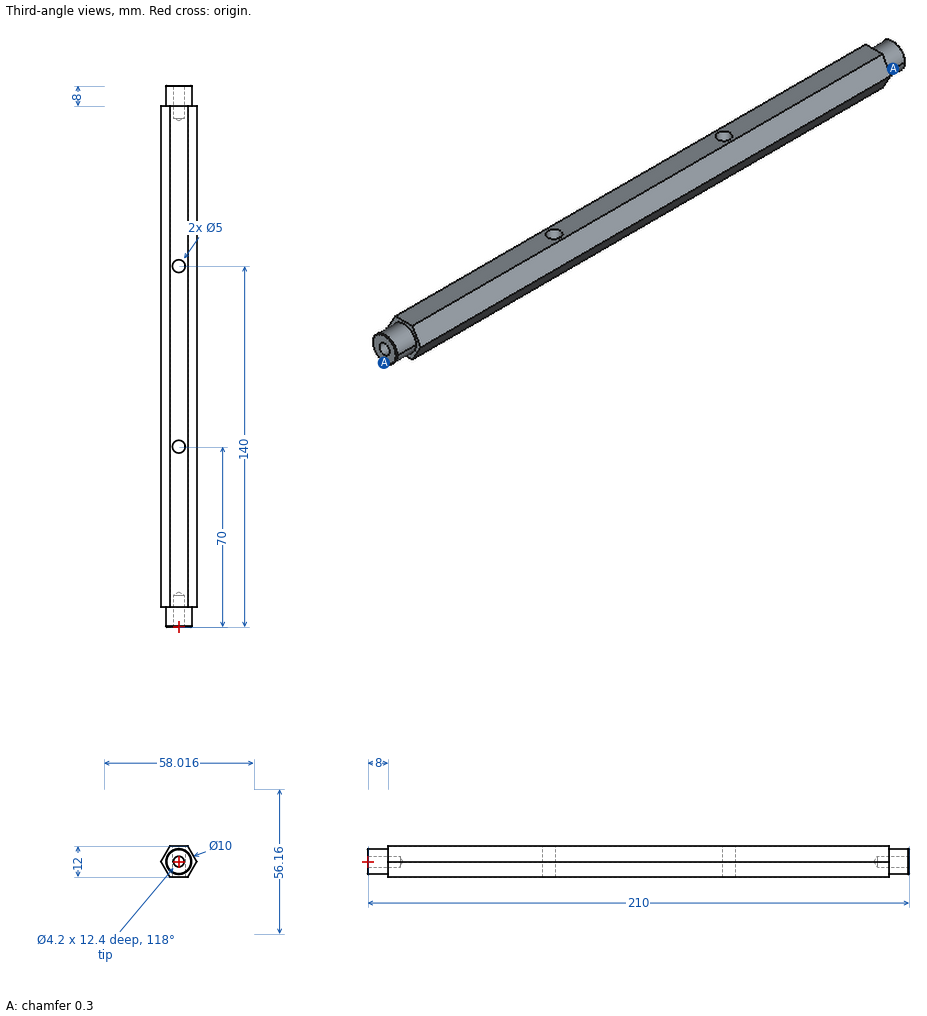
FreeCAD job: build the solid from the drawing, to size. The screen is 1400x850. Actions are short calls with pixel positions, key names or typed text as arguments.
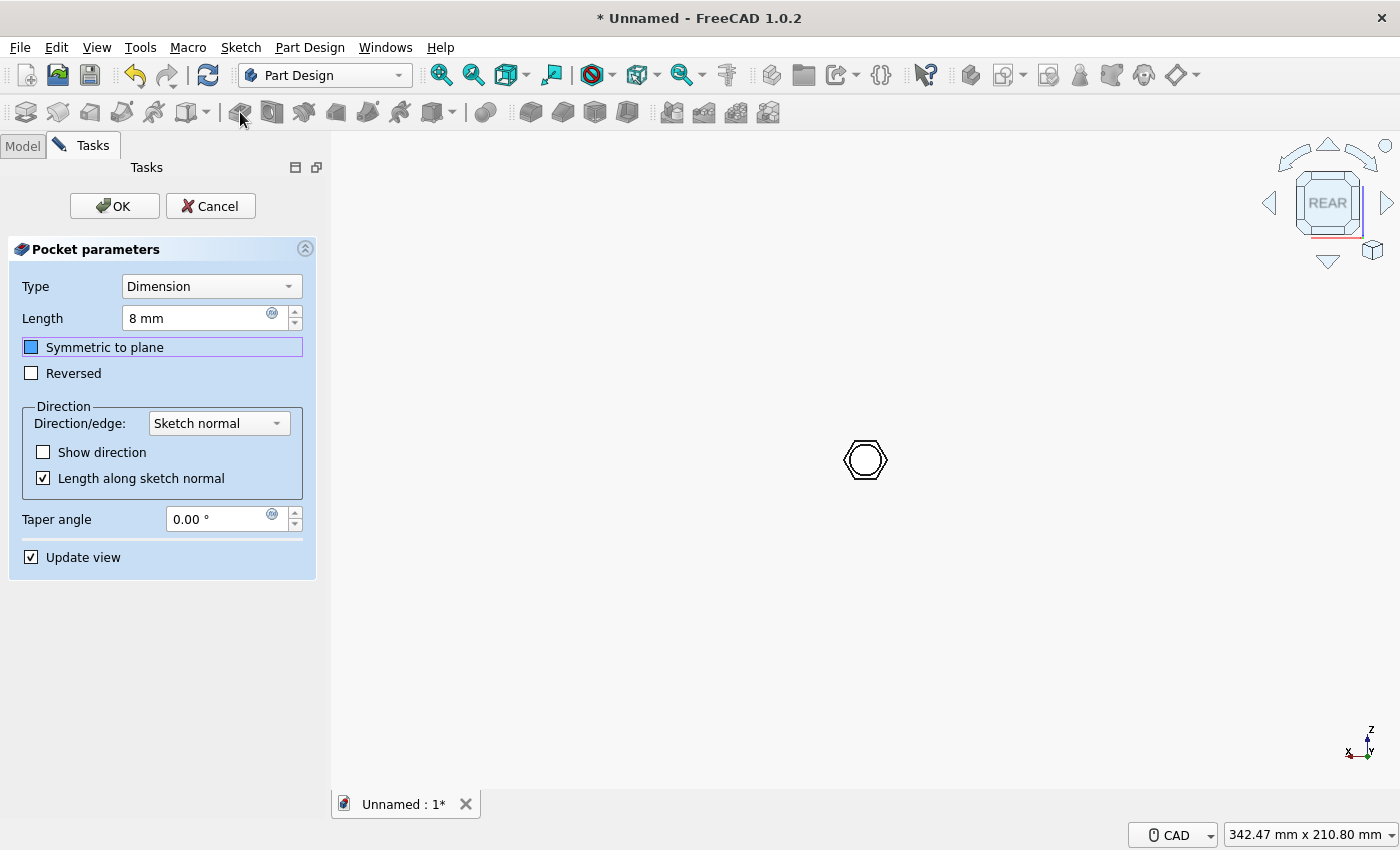
click(115, 206)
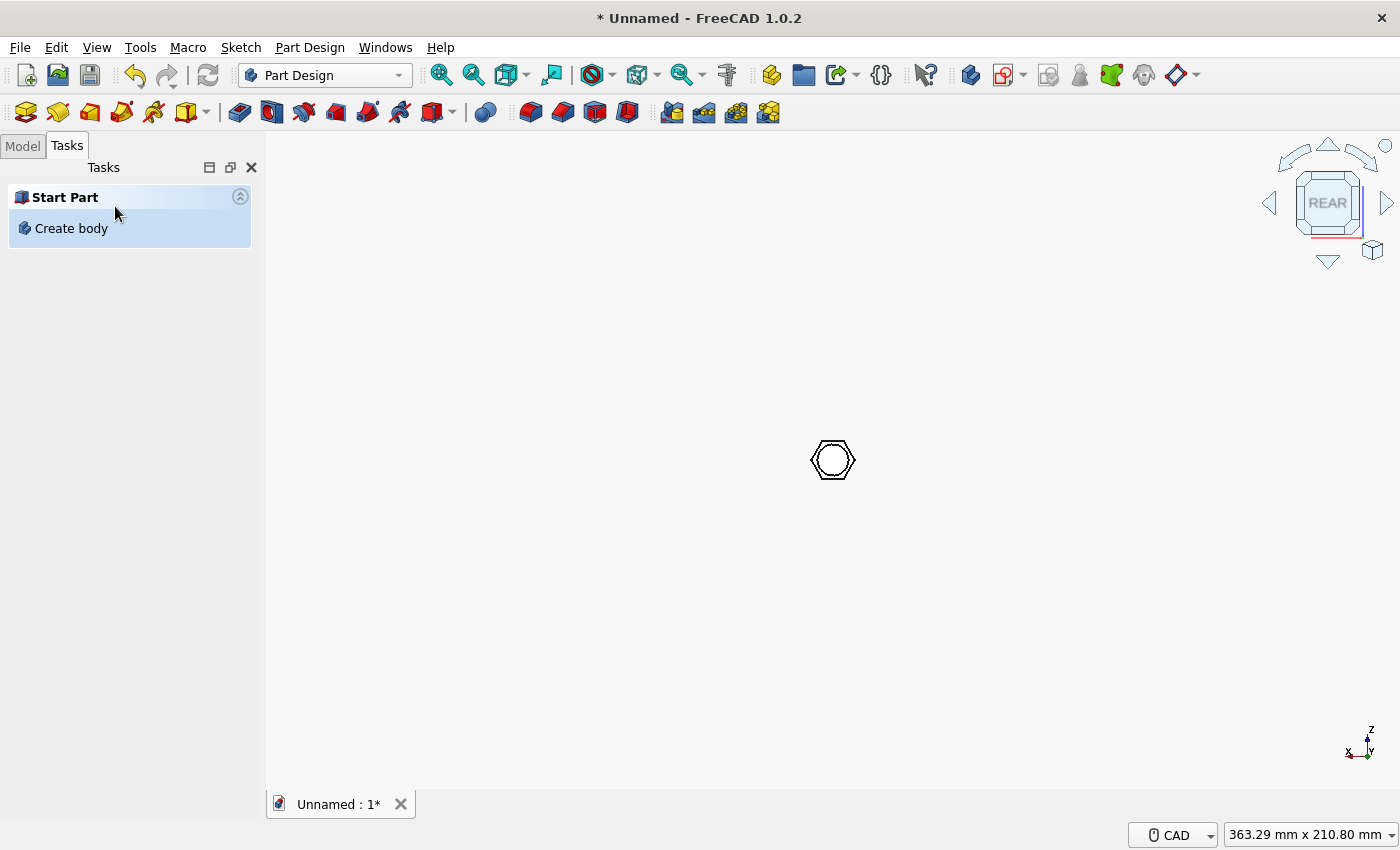
click(442, 76)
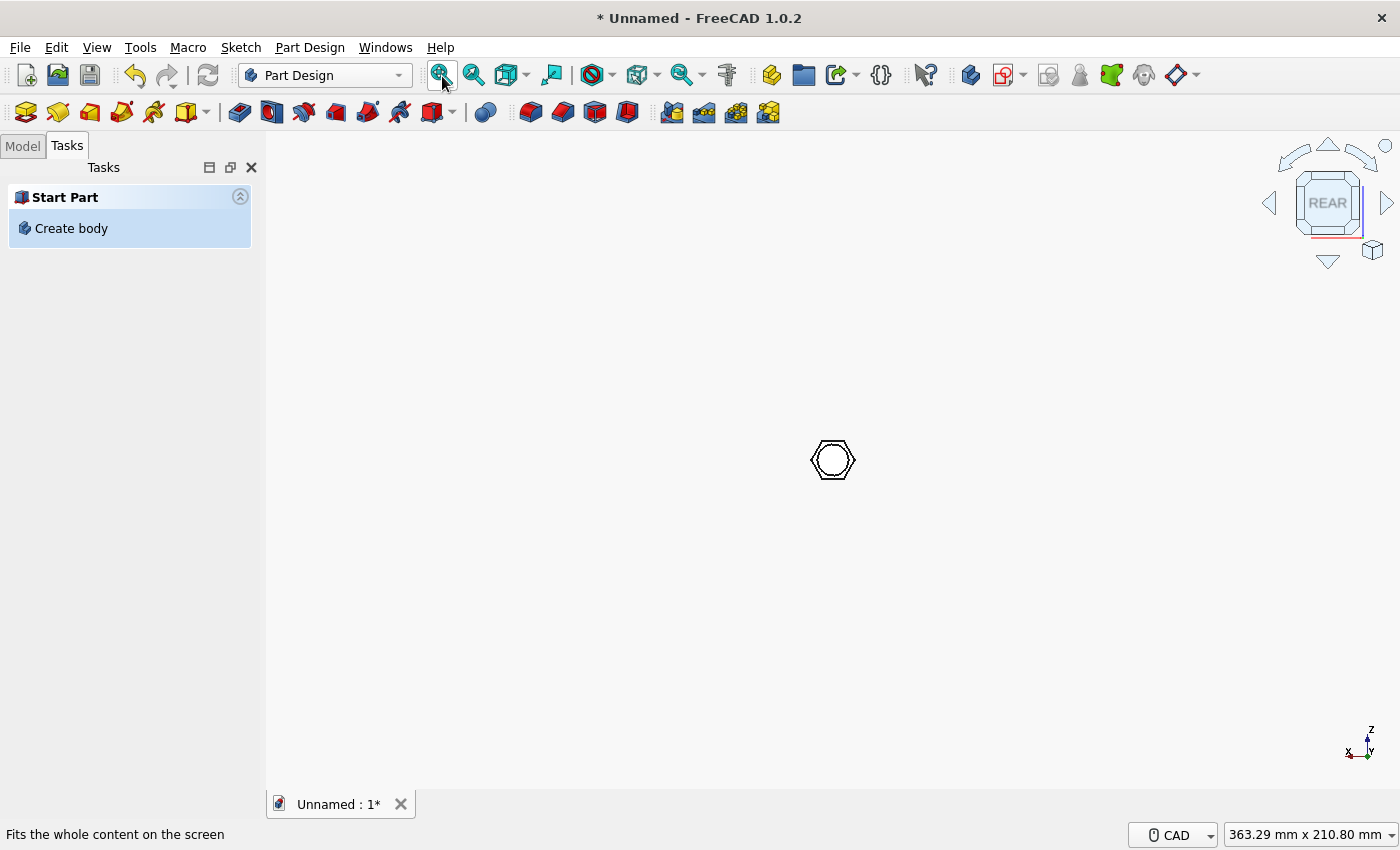
click(1004, 76)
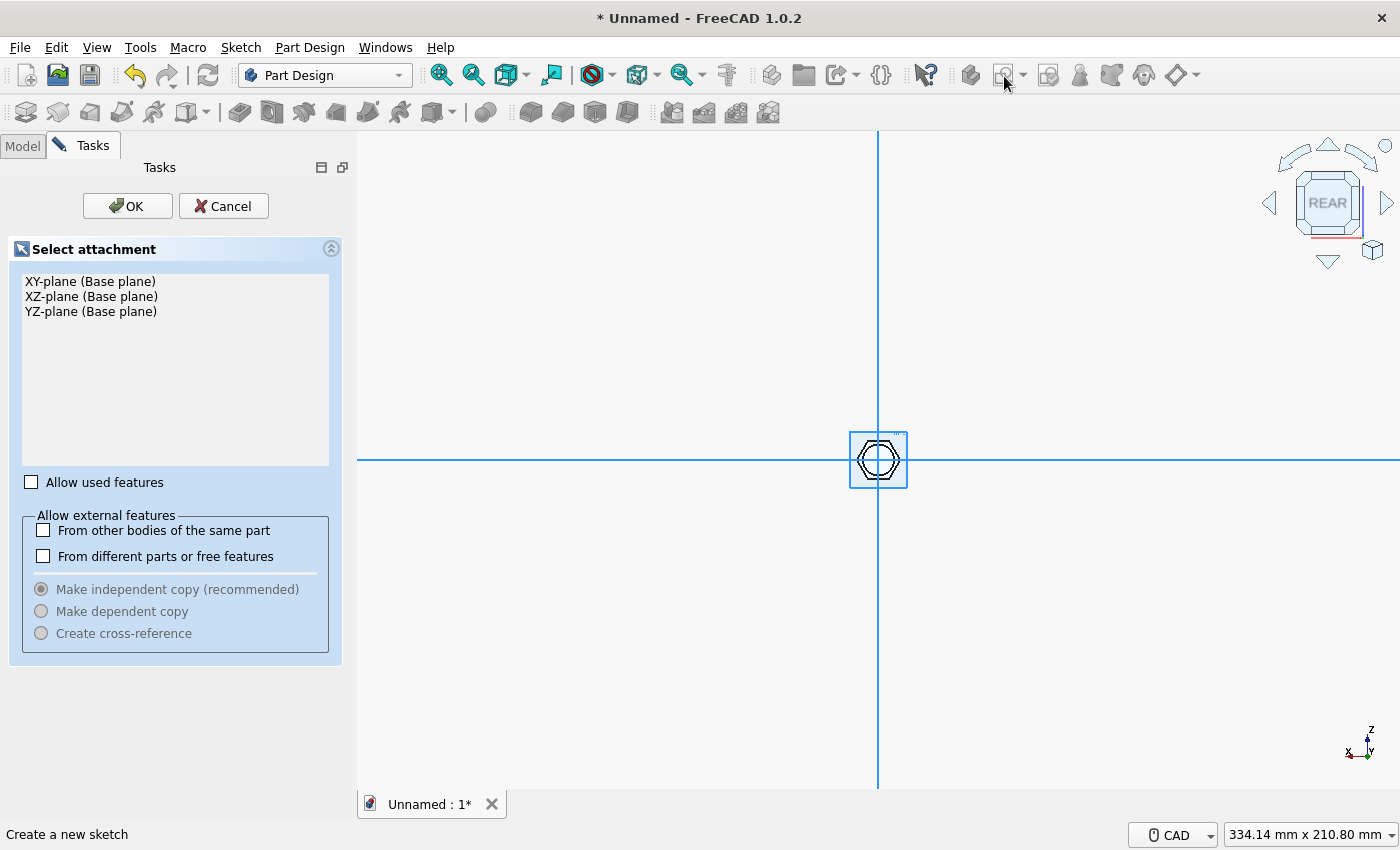
click(82, 296)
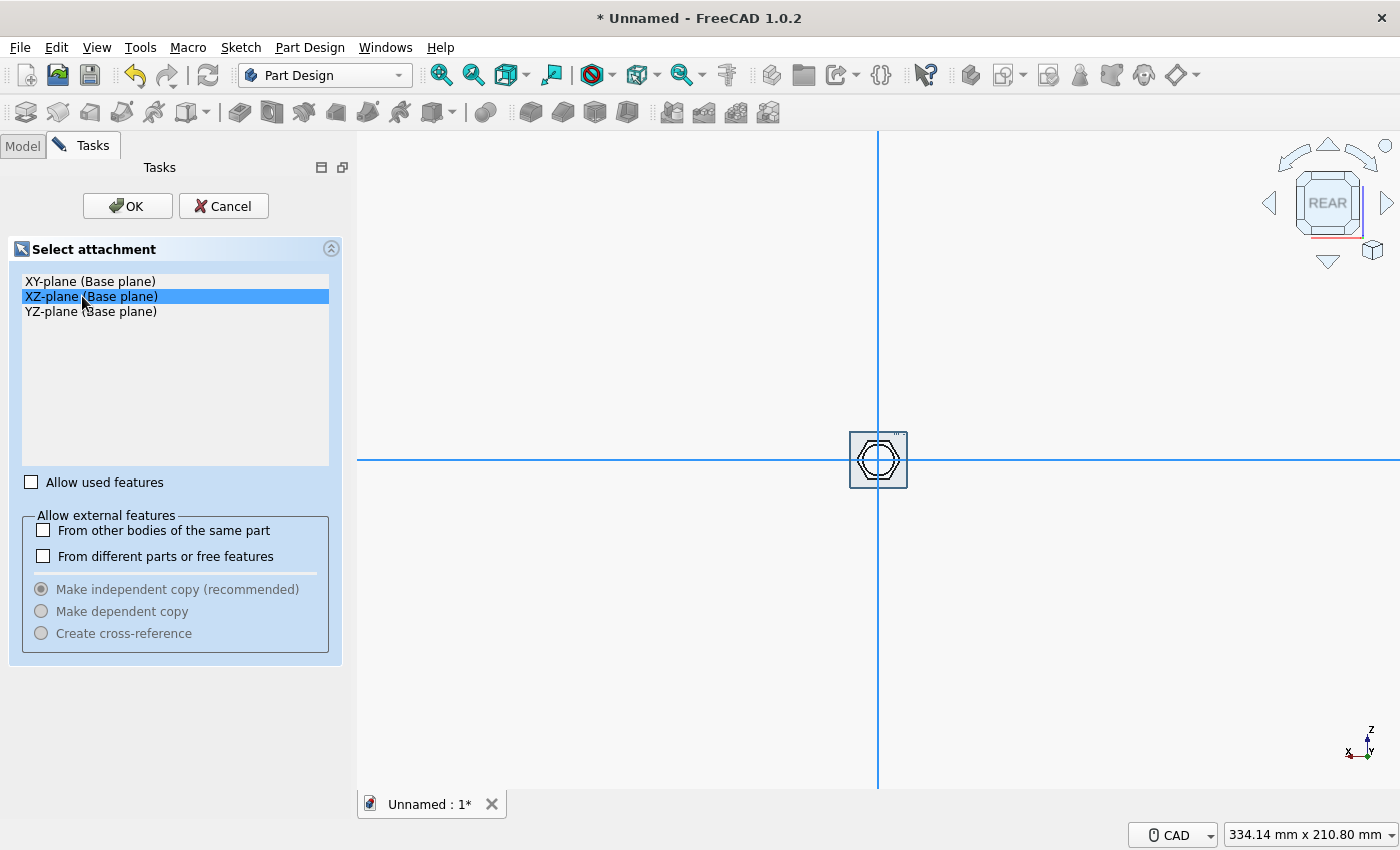
click(128, 206)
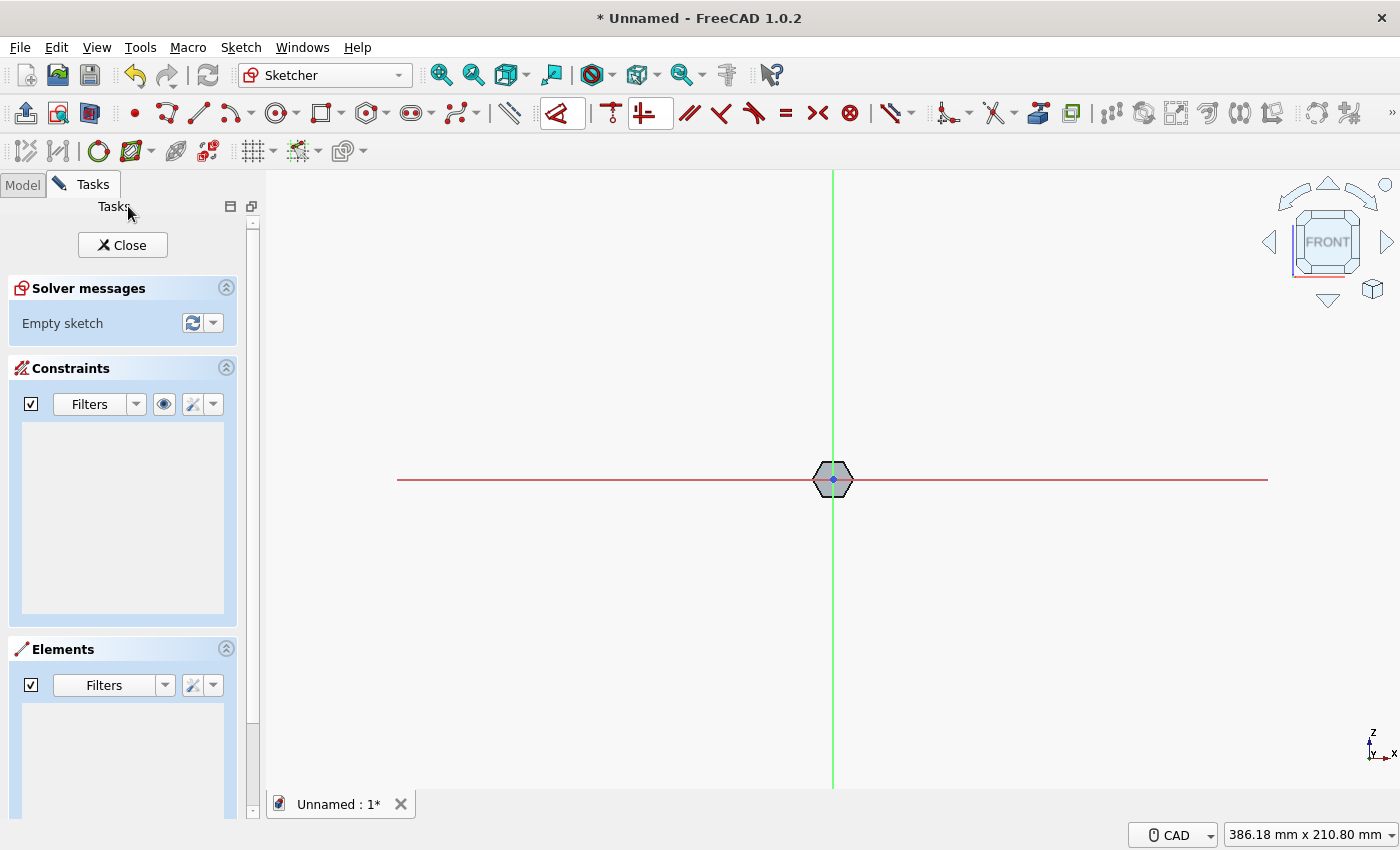
scroll(889, 480, up, 4)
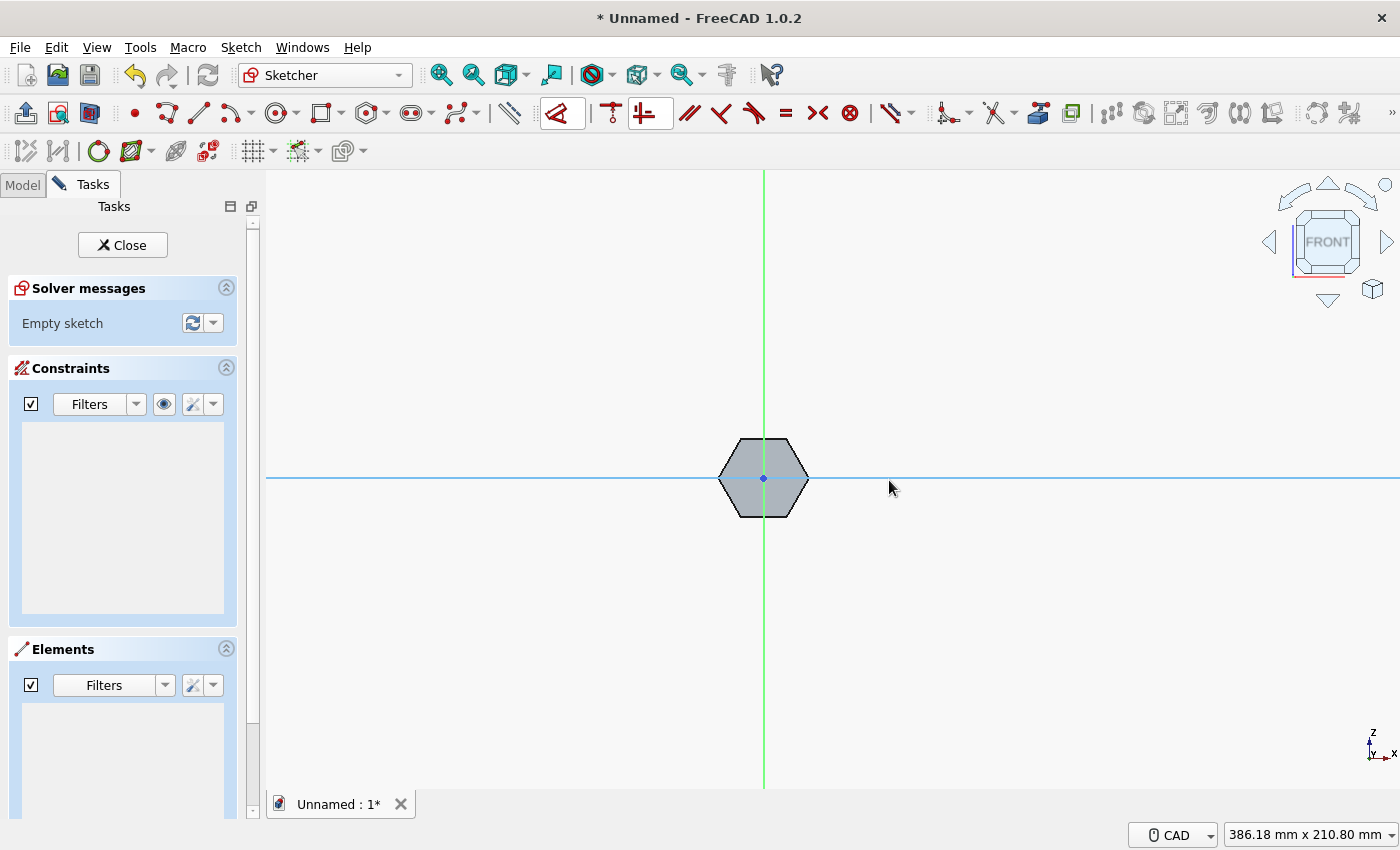
key(g)
key(v)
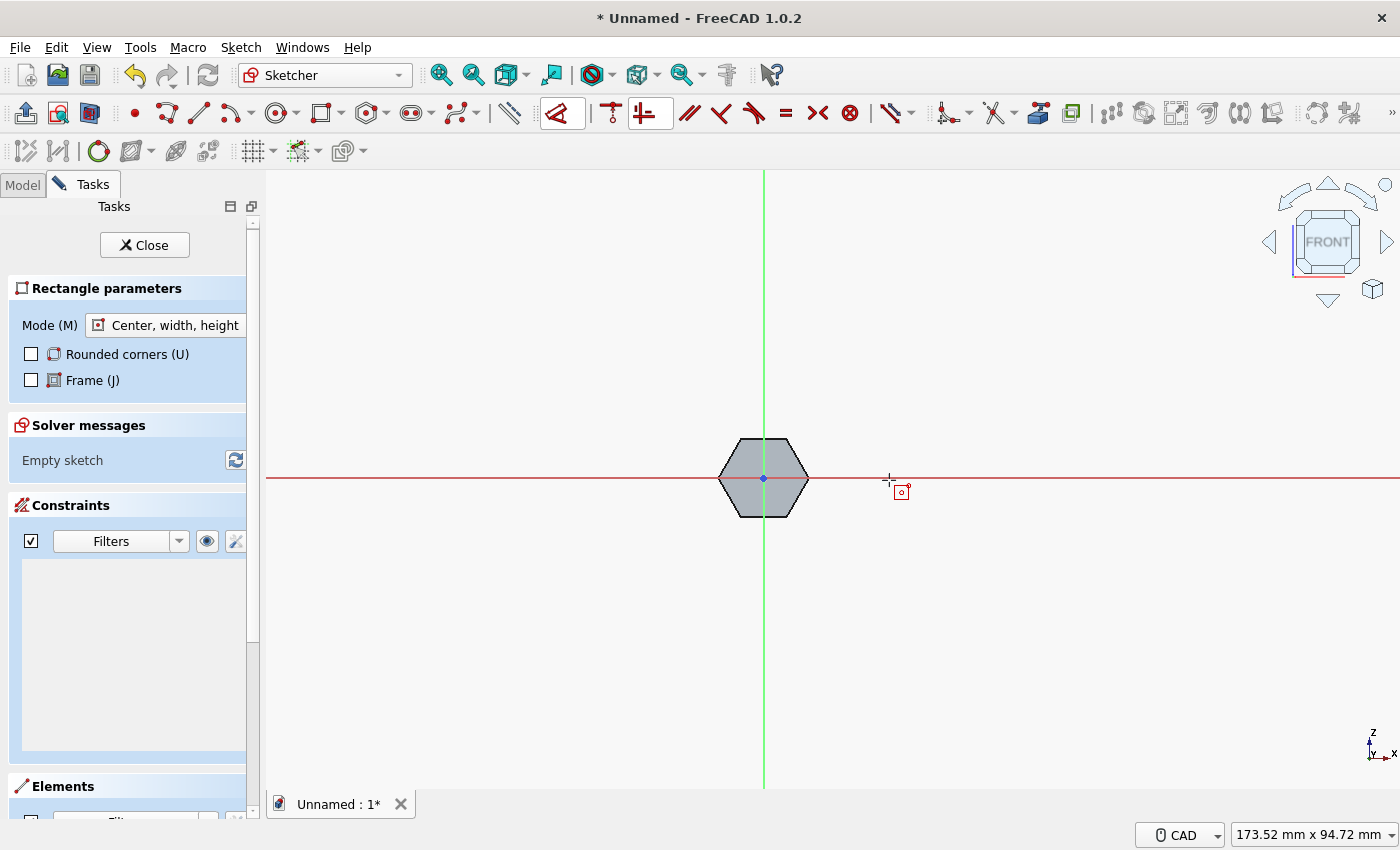
click(764, 478)
click(953, 295)